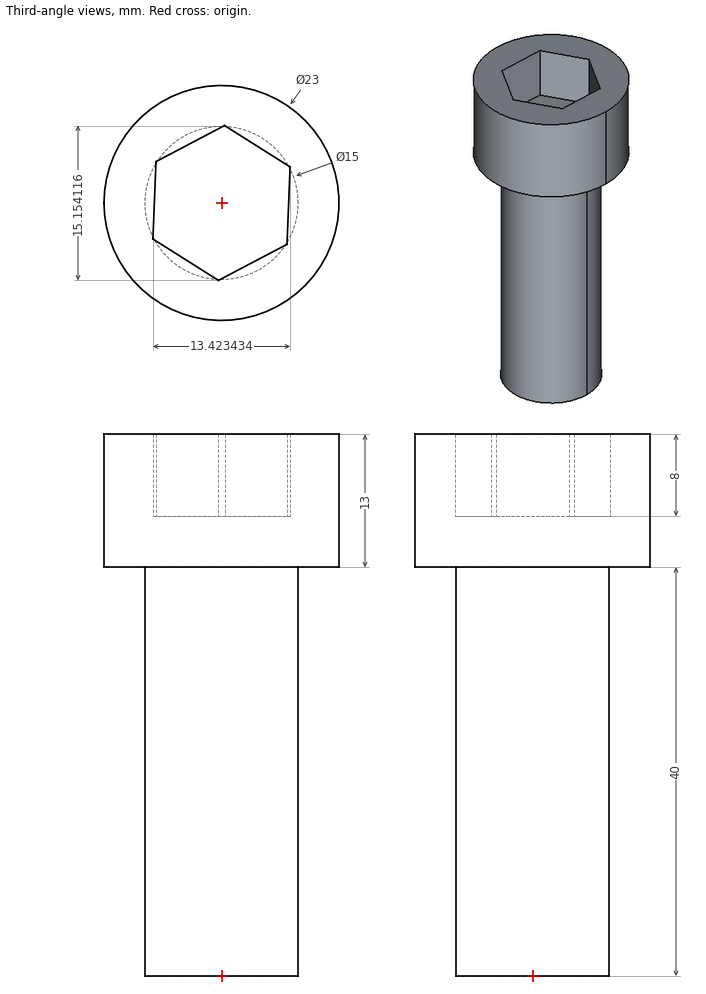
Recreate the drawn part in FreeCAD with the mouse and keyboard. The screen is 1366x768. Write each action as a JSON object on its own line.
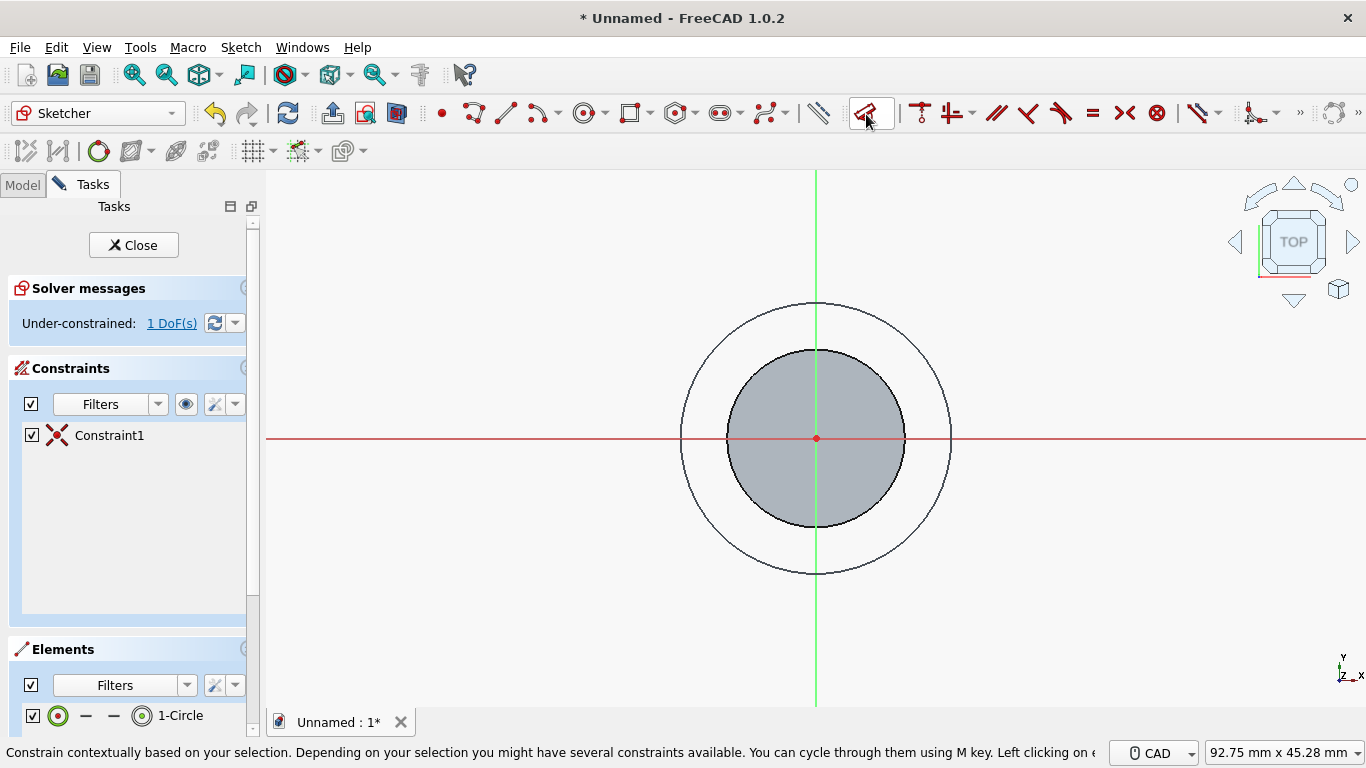
{"action": "left_click", "coordinate": [911, 342]}
{"action": "left_click", "coordinate": [933, 319]}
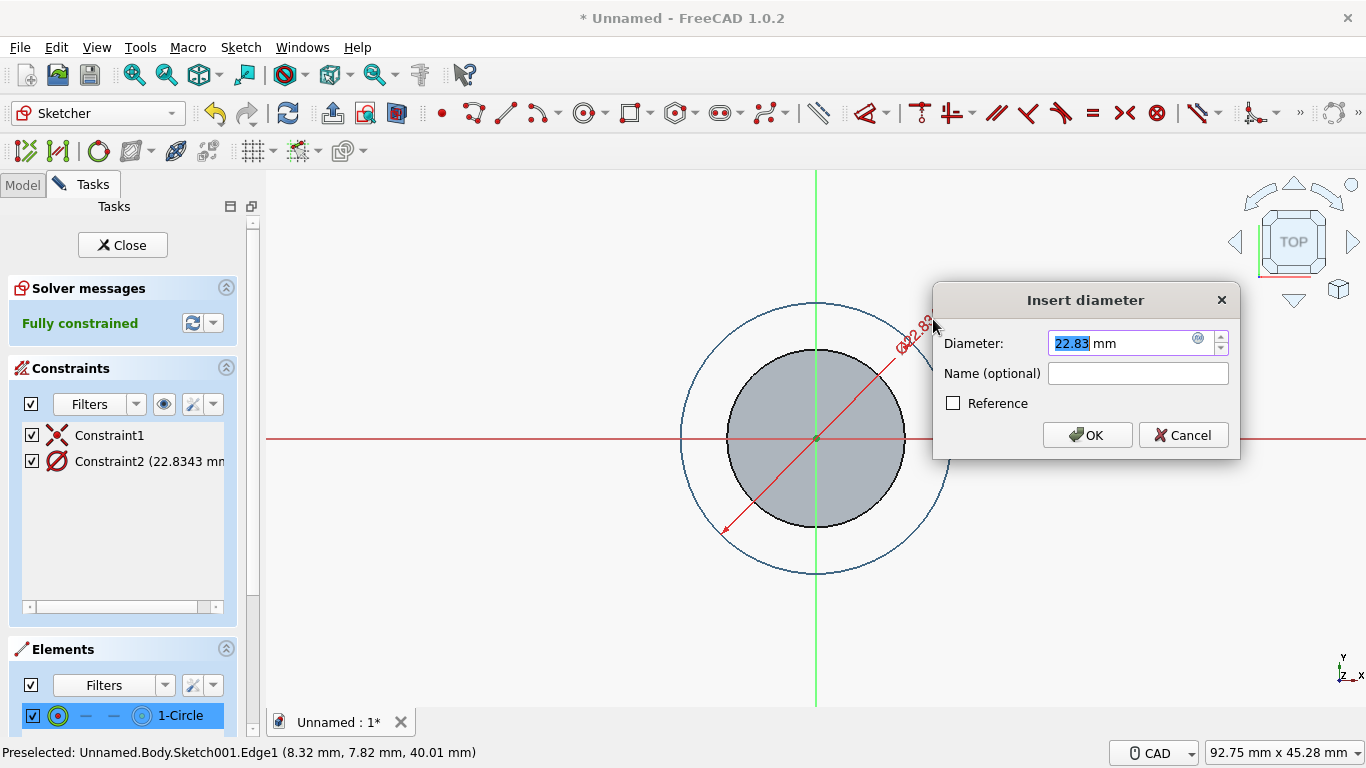
{"action": "type", "text": "23"}
{"action": "key", "text": "Return"}
{"action": "key", "text": "Escape"}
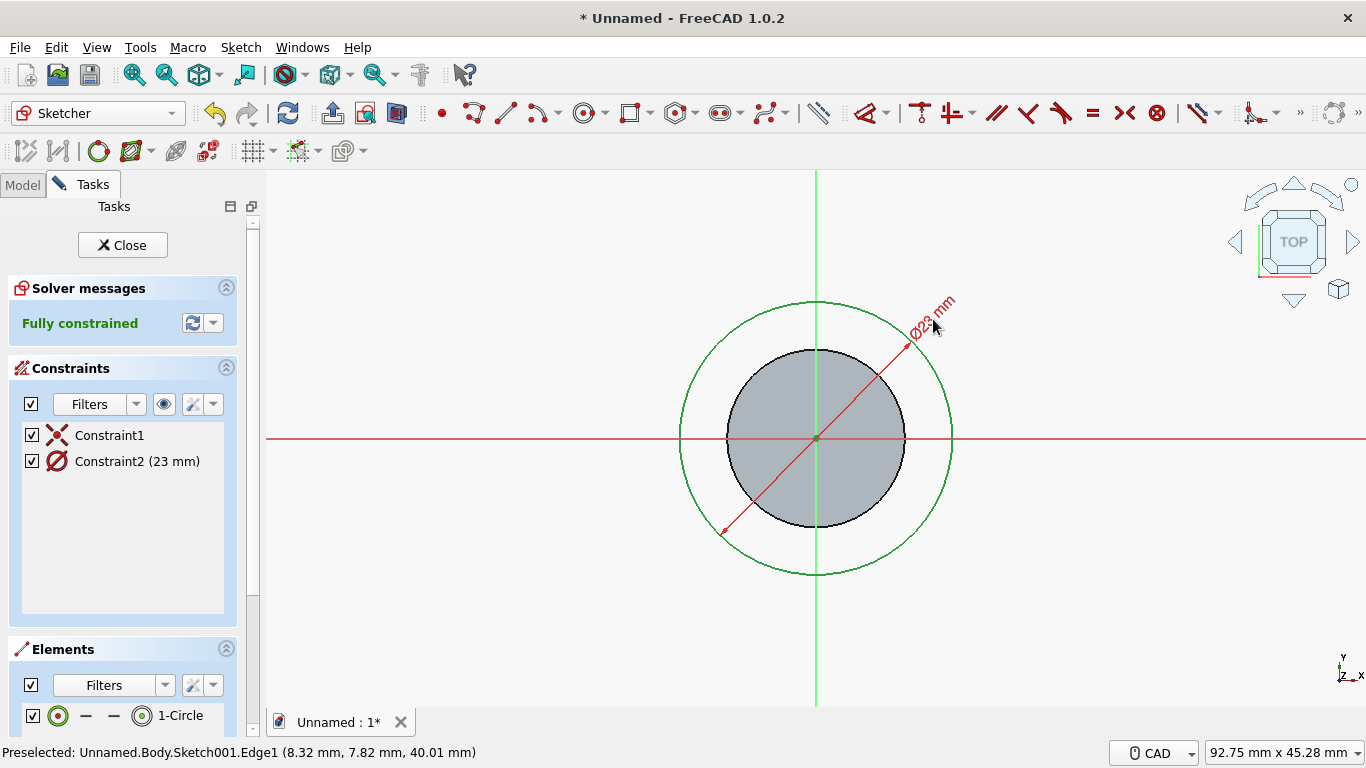
{"action": "left_click", "coordinate": [123, 245]}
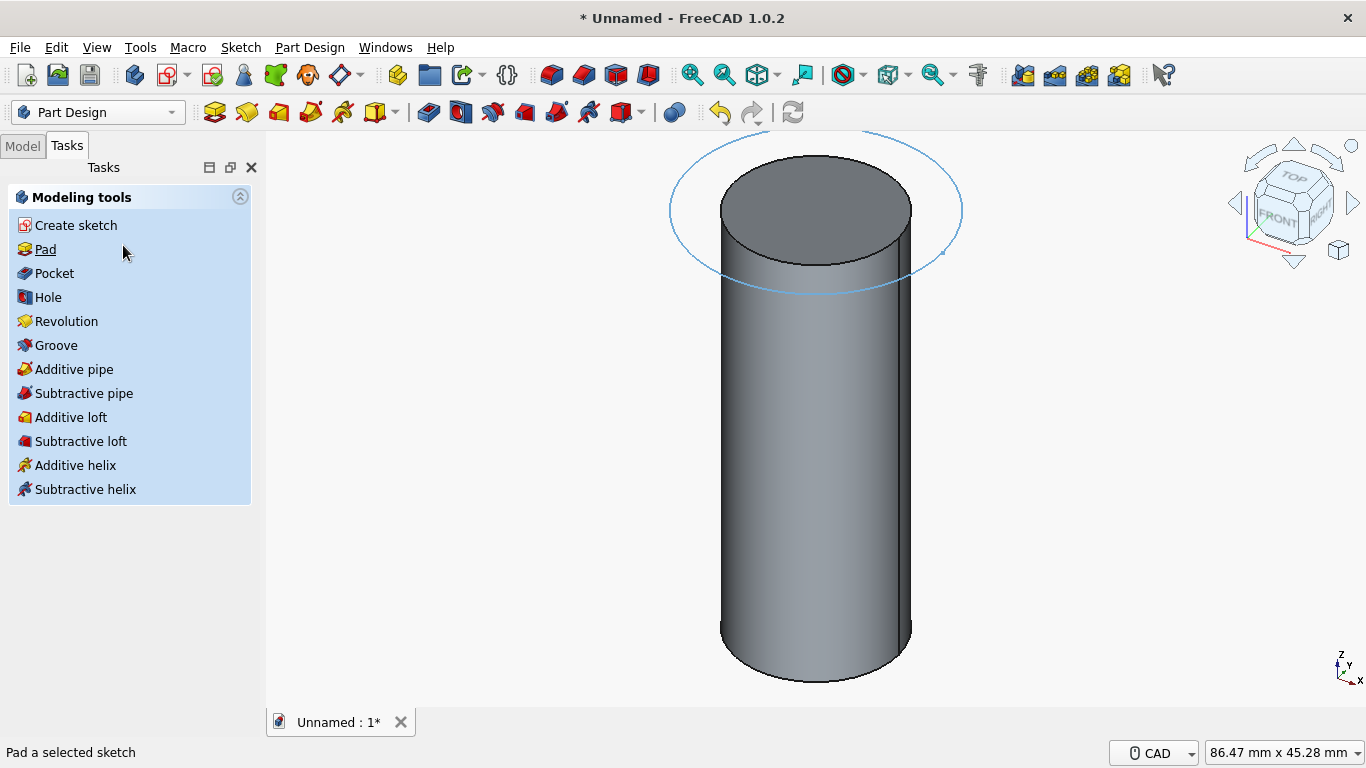
{"action": "left_click", "coordinate": [216, 112]}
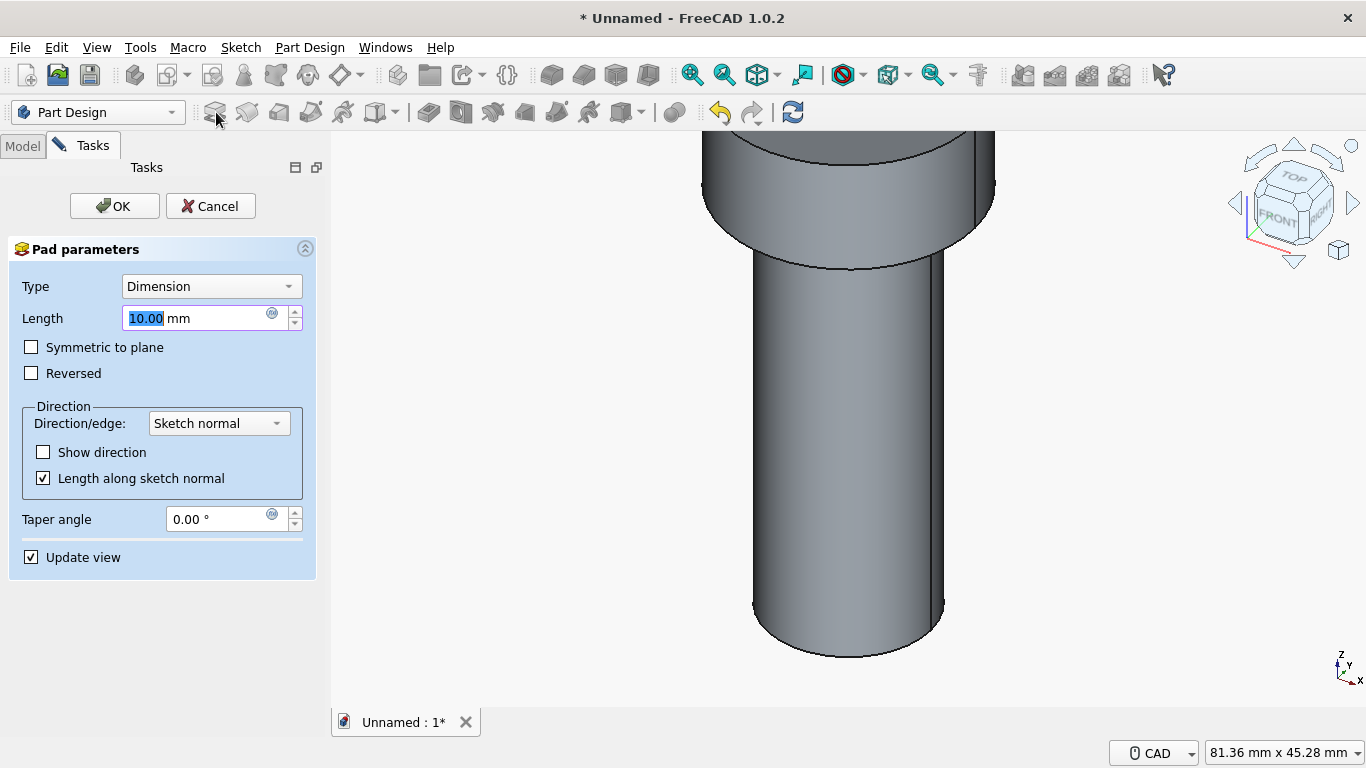
{"action": "type", "text": "13"}
{"action": "key", "text": "Tab"}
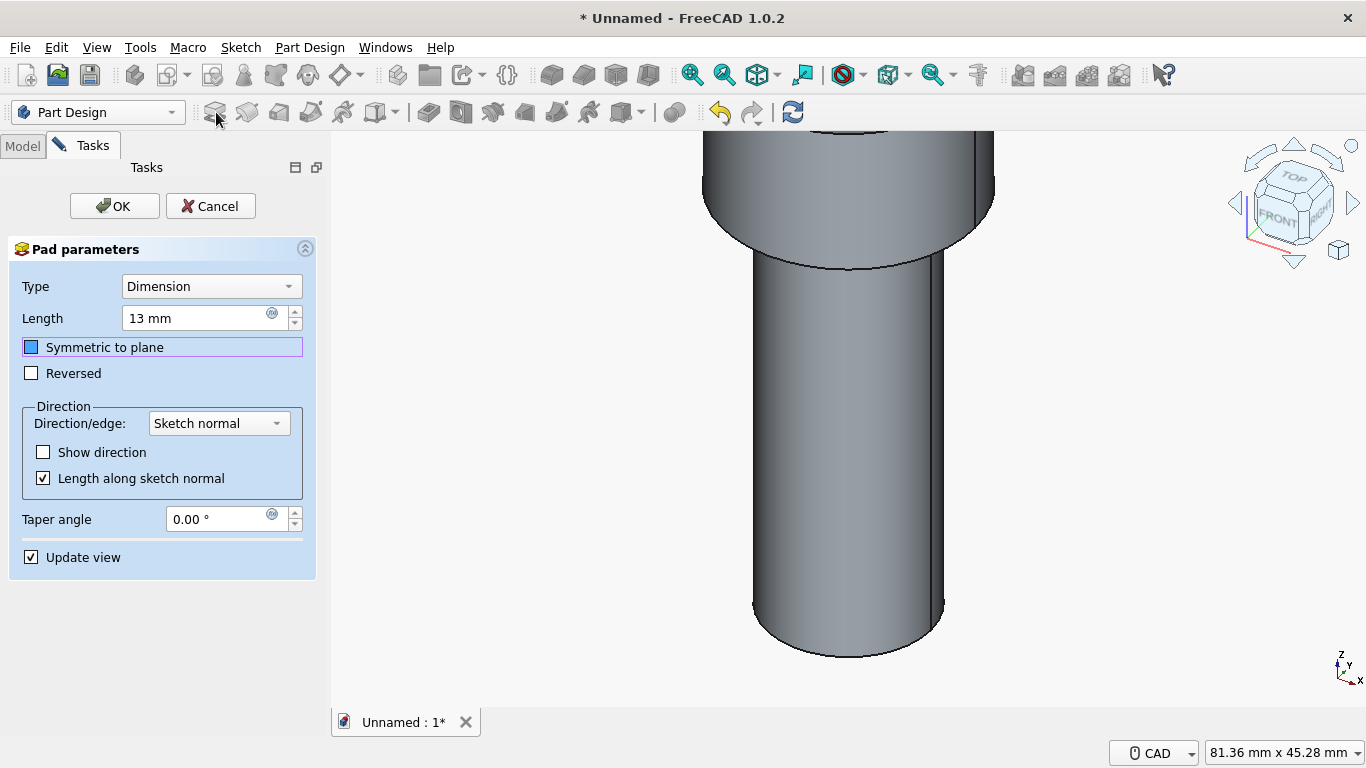
{"action": "left_click", "coordinate": [115, 206]}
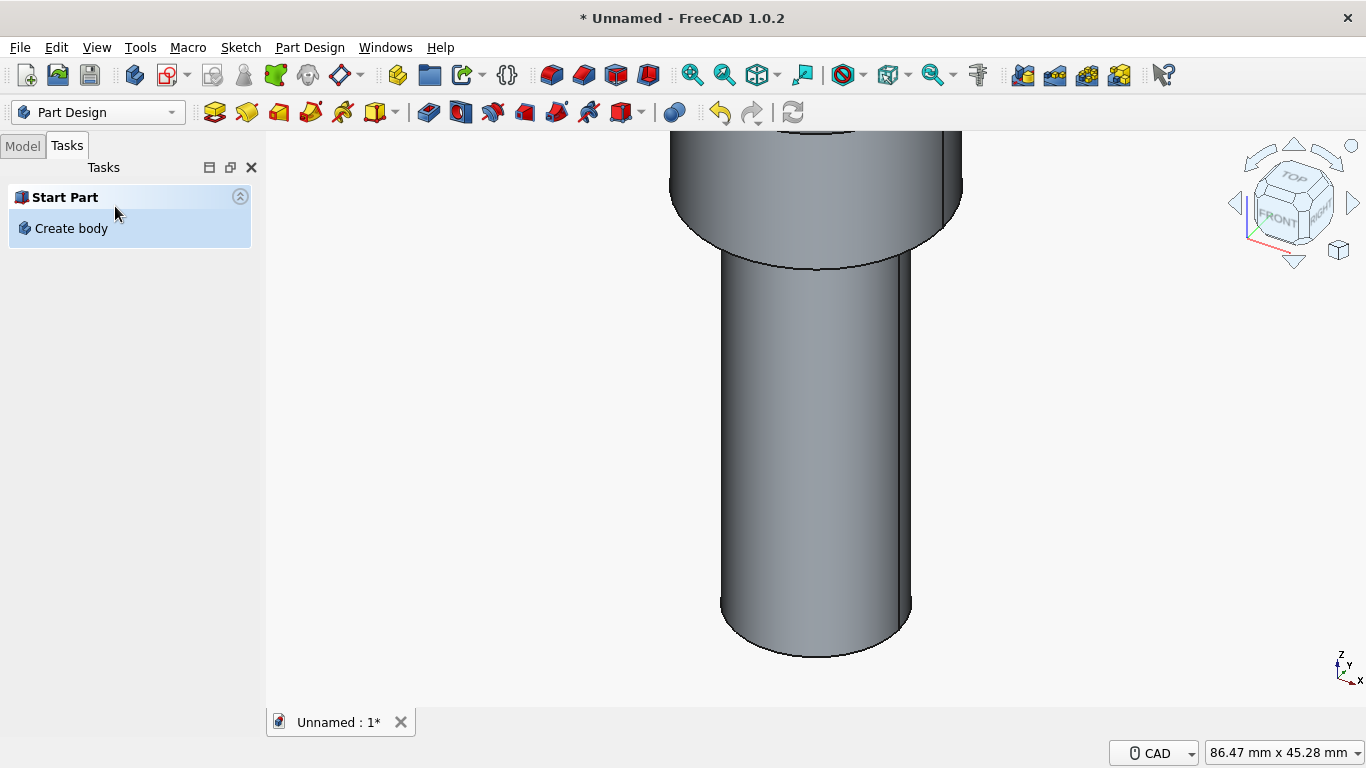
{"action": "left_click", "coordinate": [694, 76]}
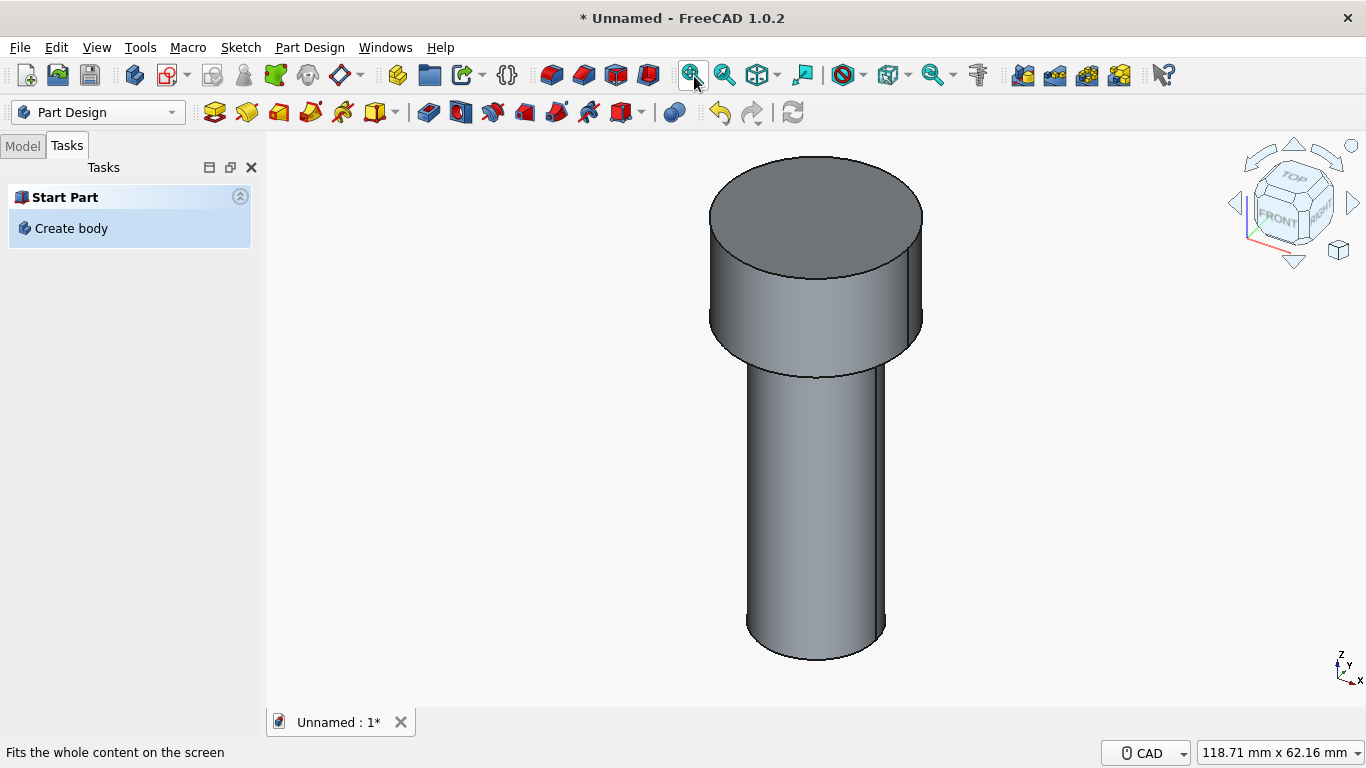
{"action": "left_click", "coordinate": [816, 217]}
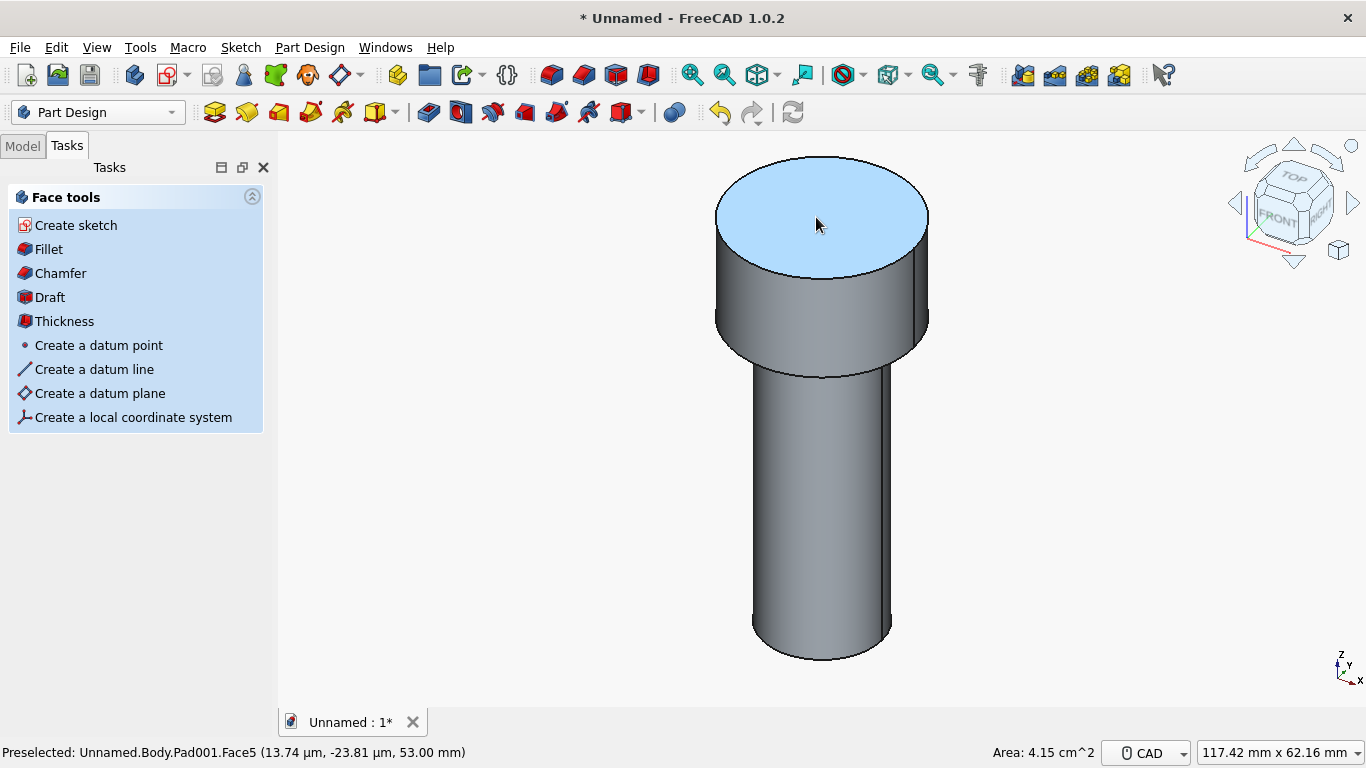
{"action": "left_click", "coordinate": [168, 76]}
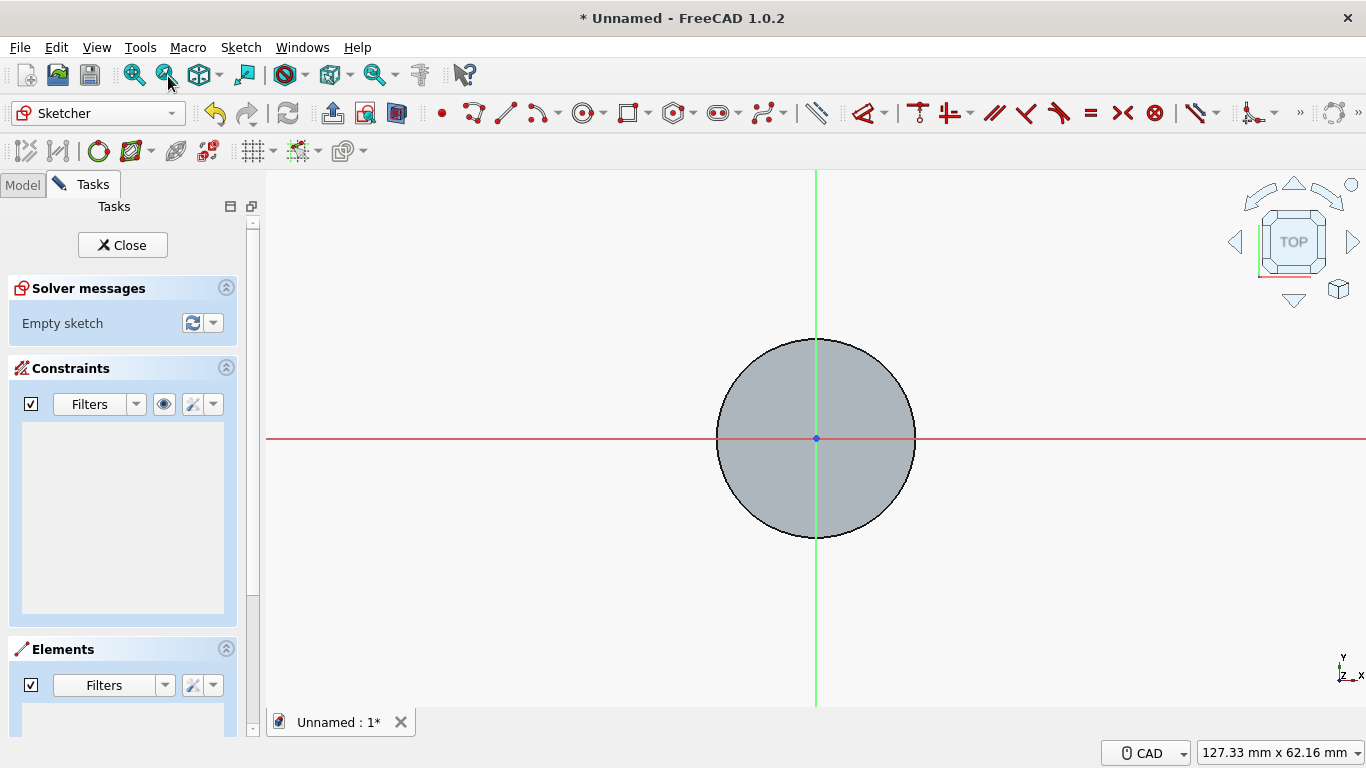
{"action": "scroll", "coordinate": [856, 439], "scroll_direction": "up", "scroll_amount": 5}